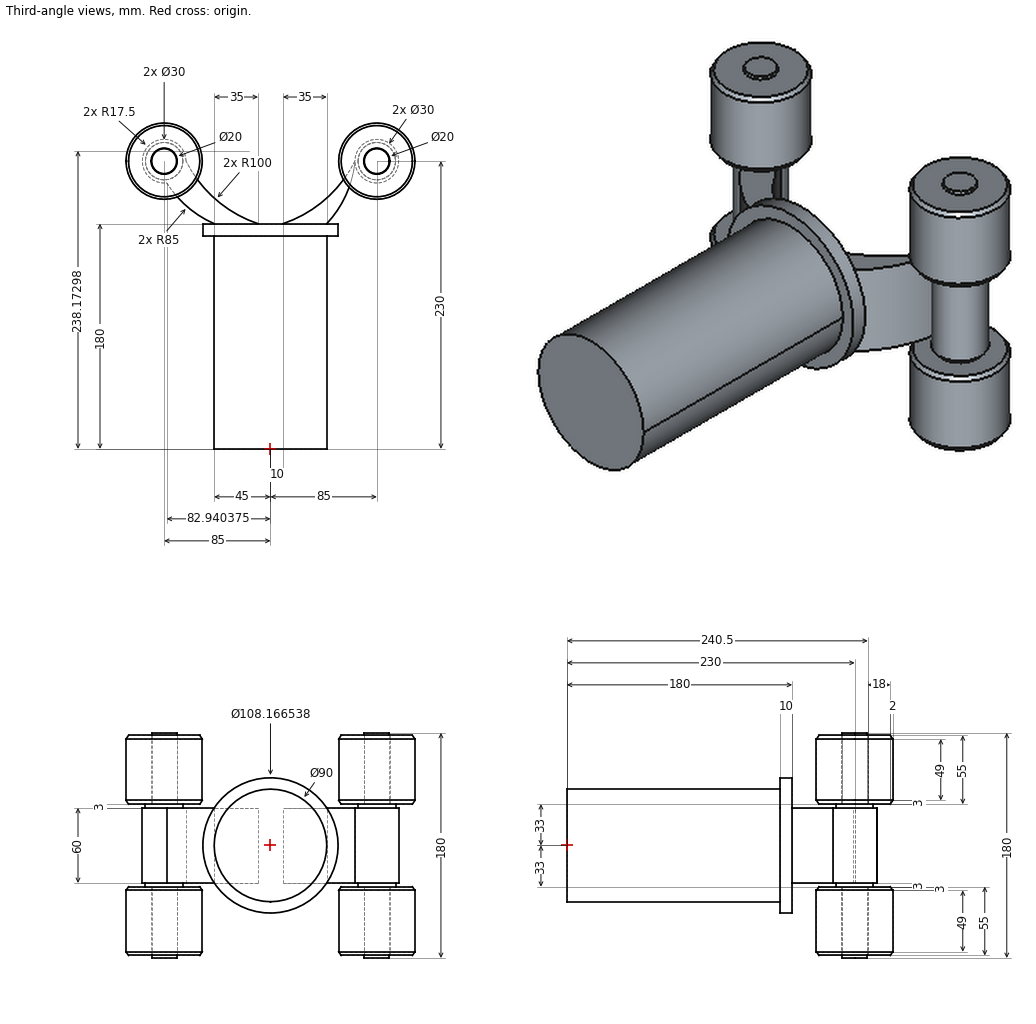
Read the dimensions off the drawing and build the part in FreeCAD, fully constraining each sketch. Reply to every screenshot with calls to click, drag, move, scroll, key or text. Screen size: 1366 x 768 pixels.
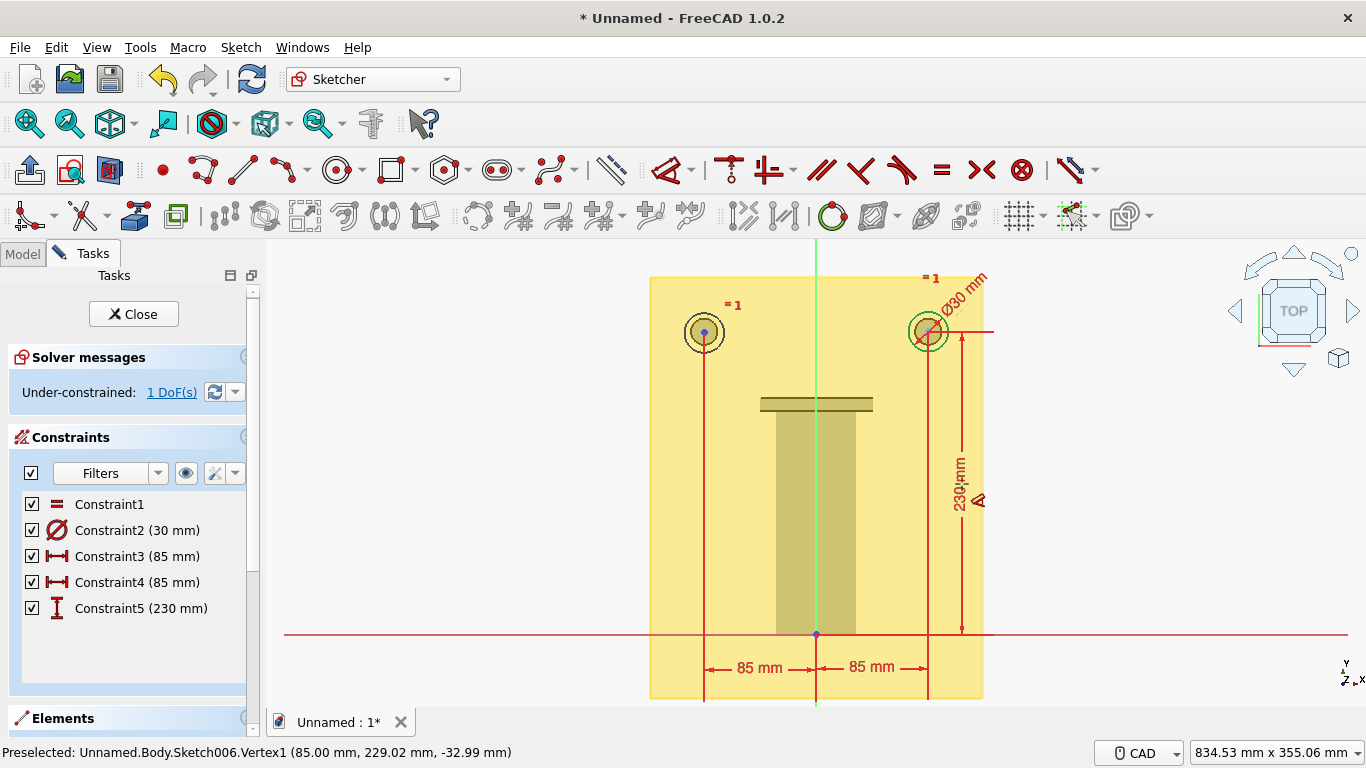
click(704, 333)
click(670, 484)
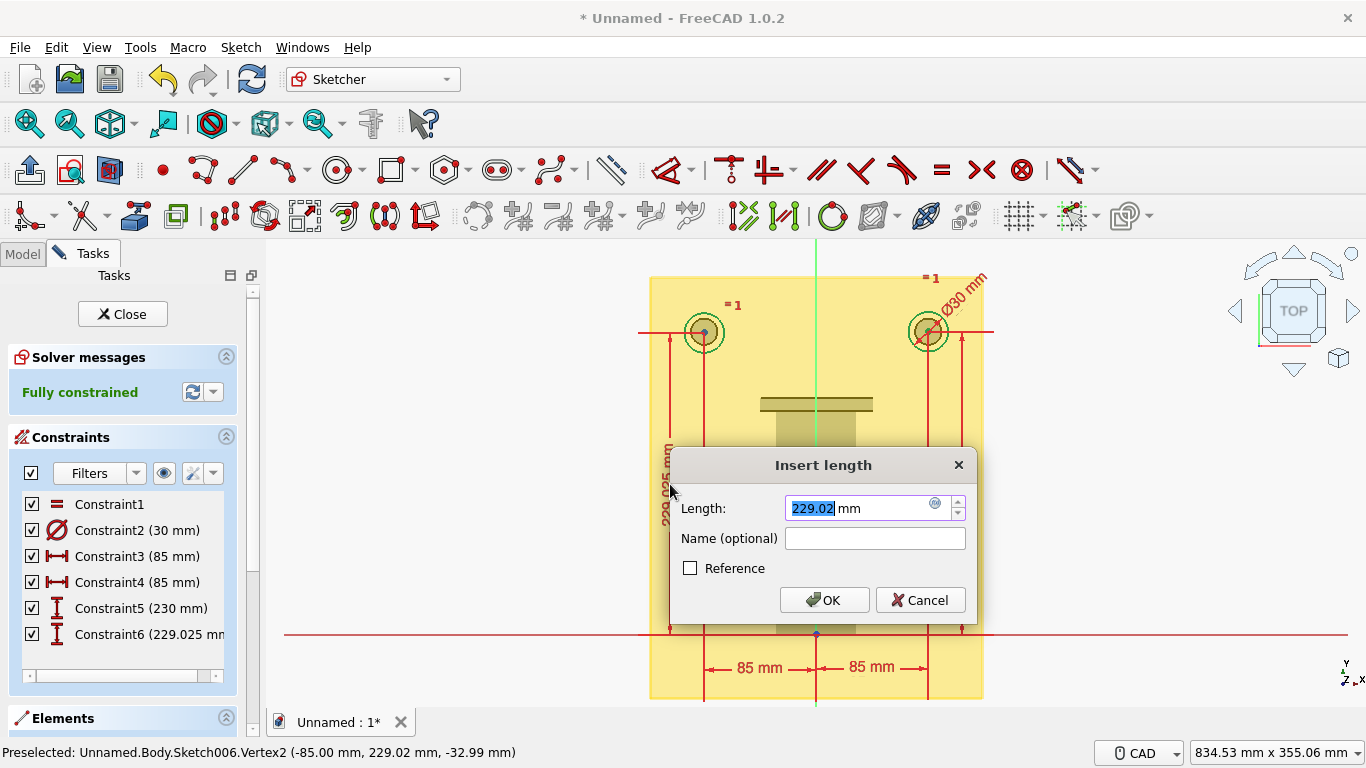
text(230)
key(Return)
key(Escape)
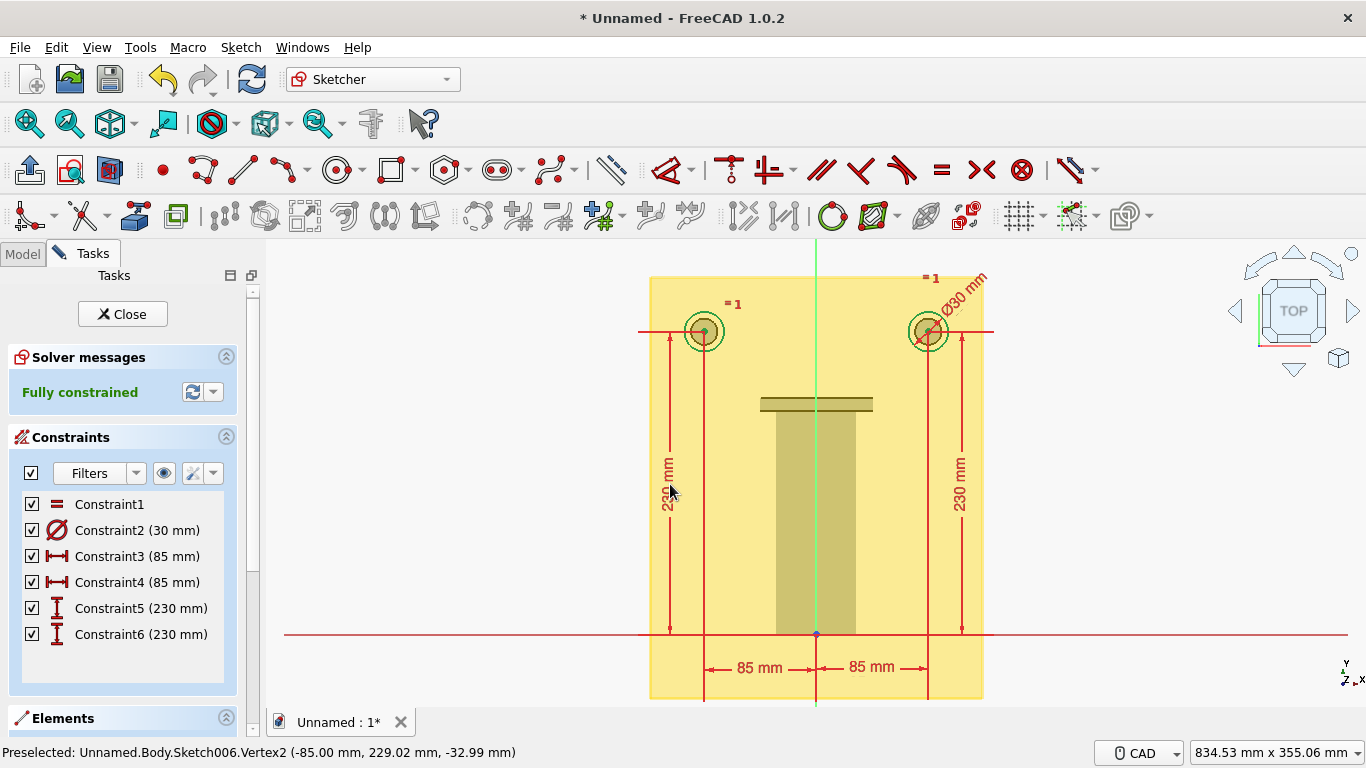
click(123, 314)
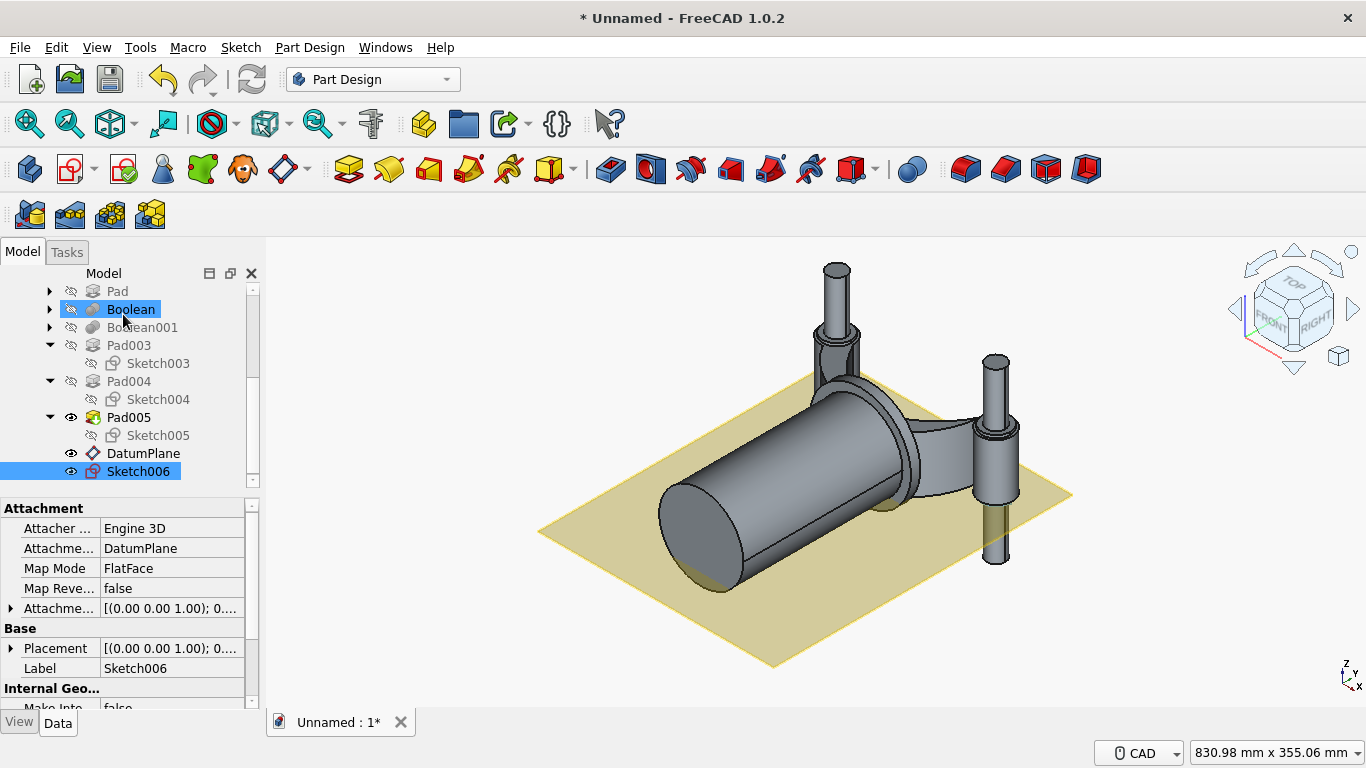
click(350, 170)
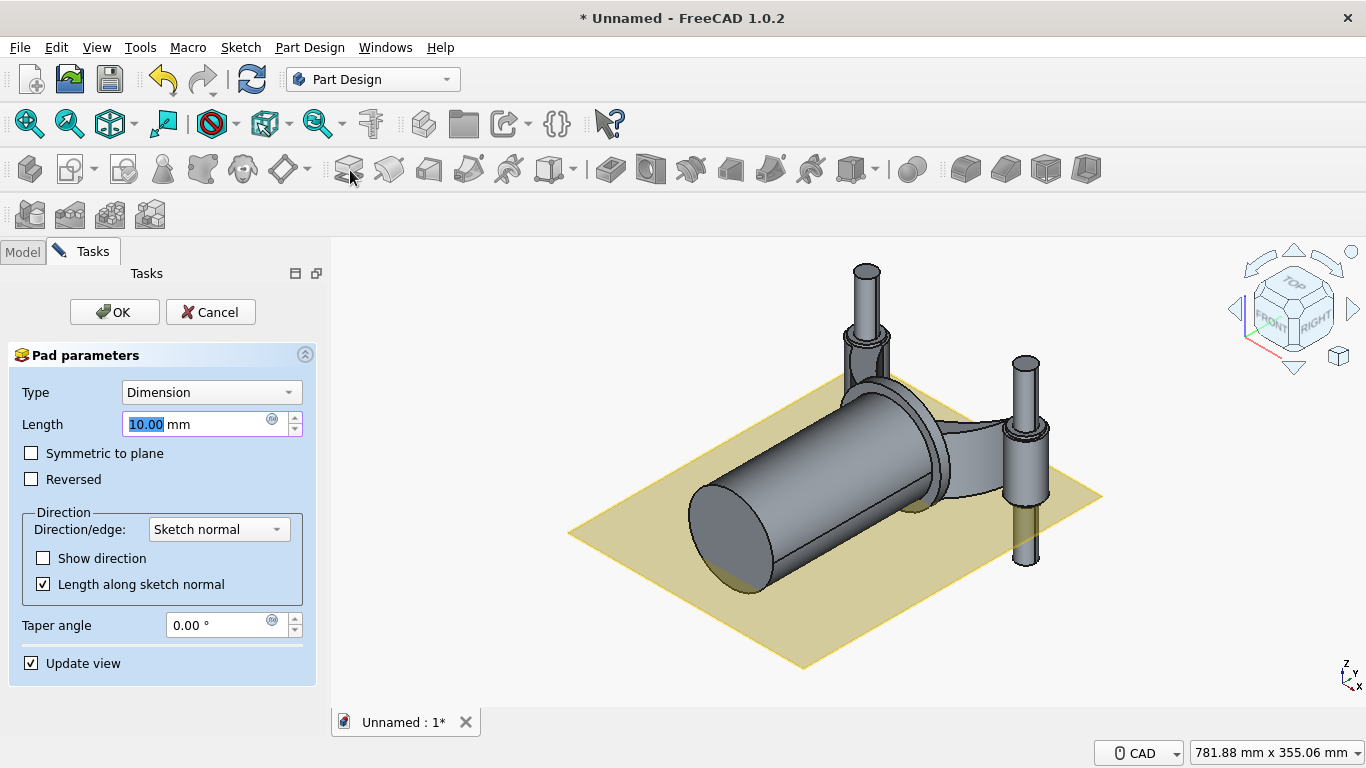
text(3)
key(Tab)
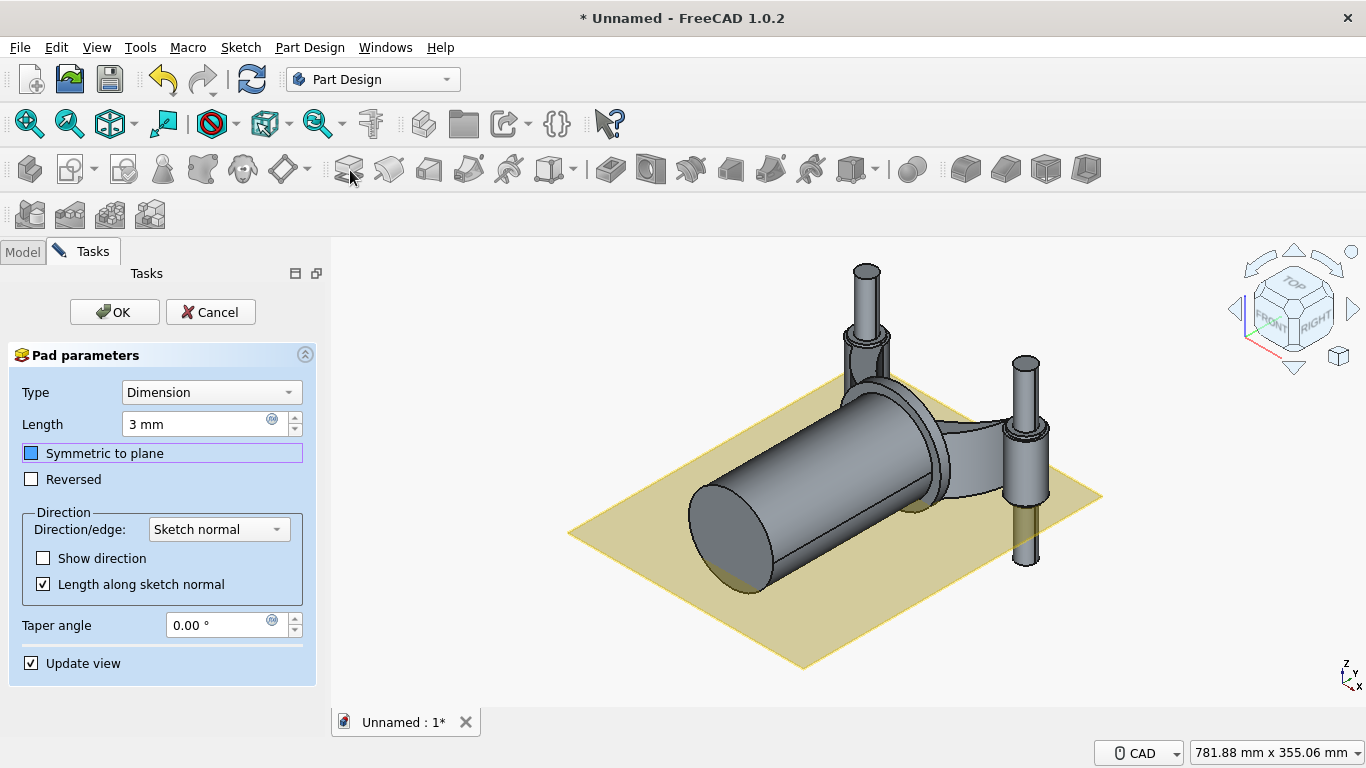
click(115, 312)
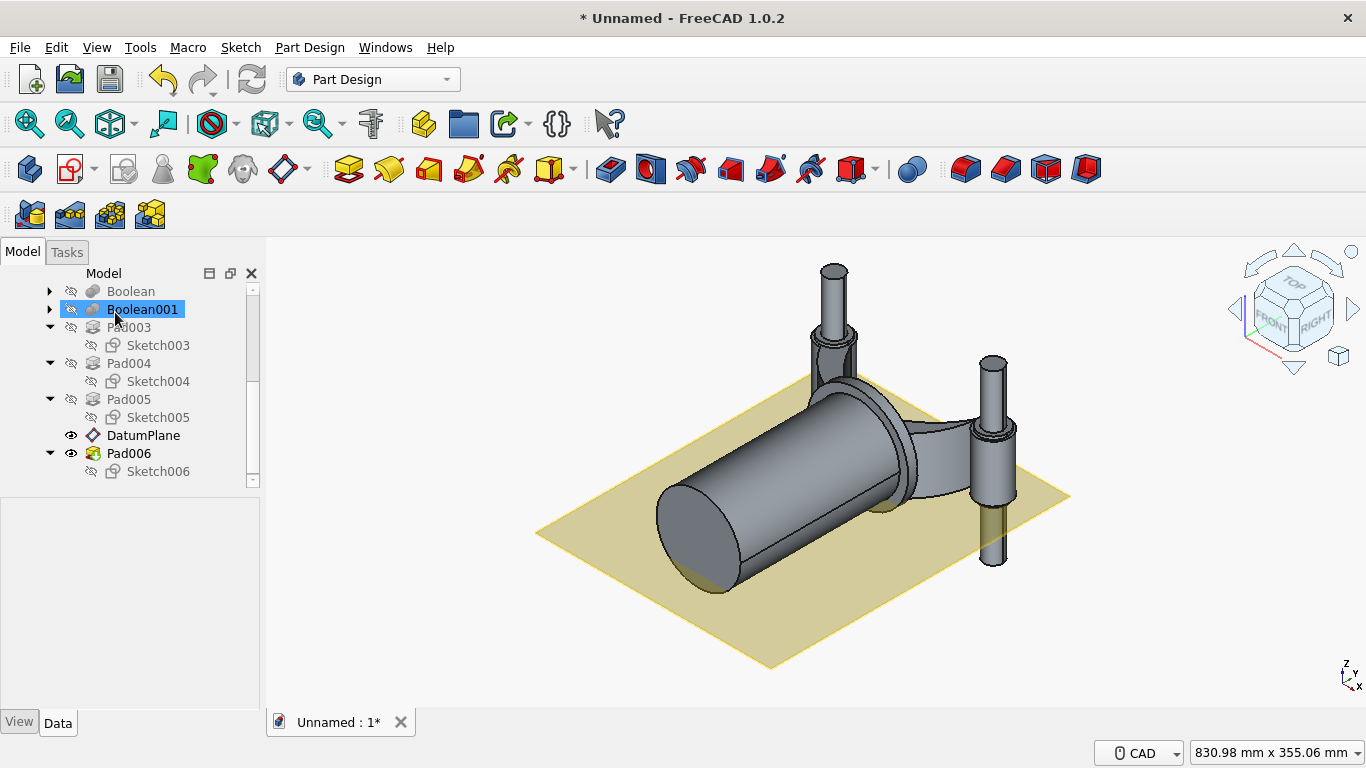
click(116, 435)
key(space)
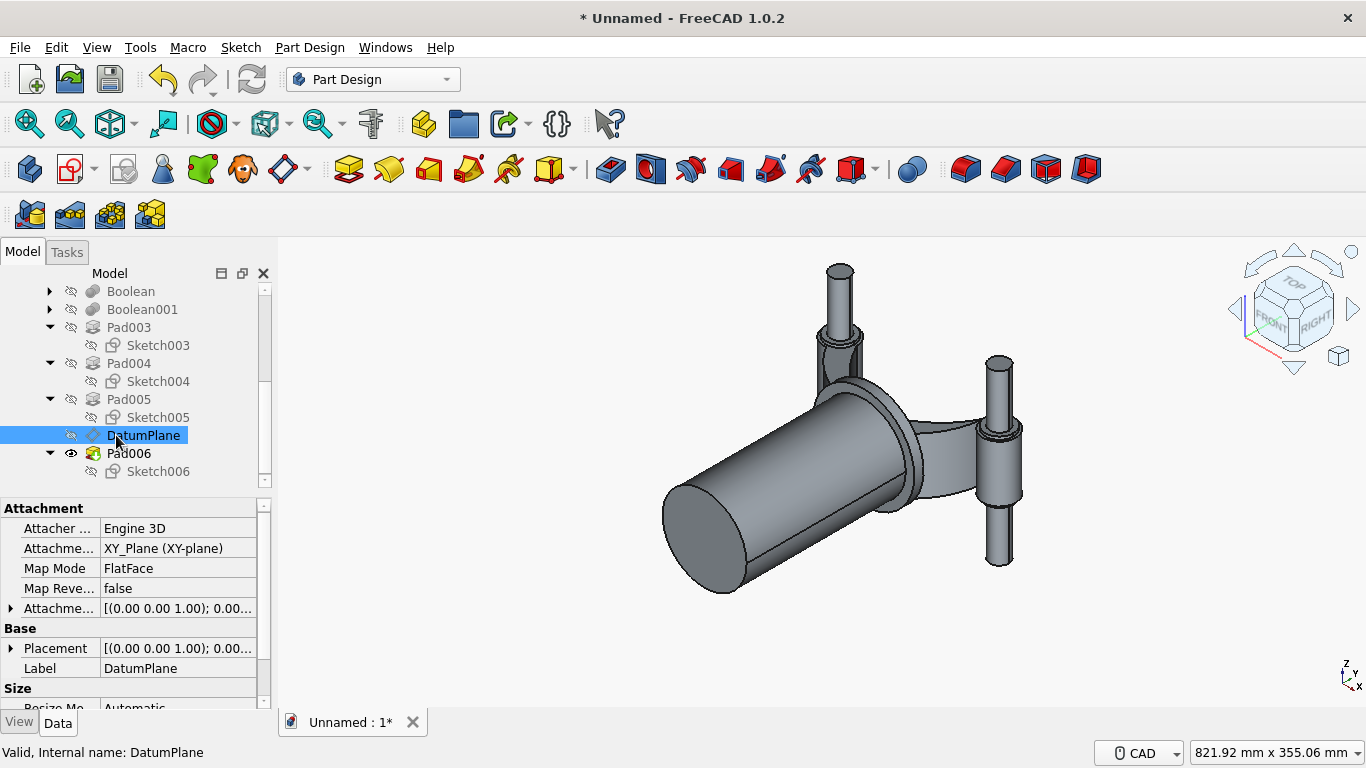
scroll(140, 377, down, 3)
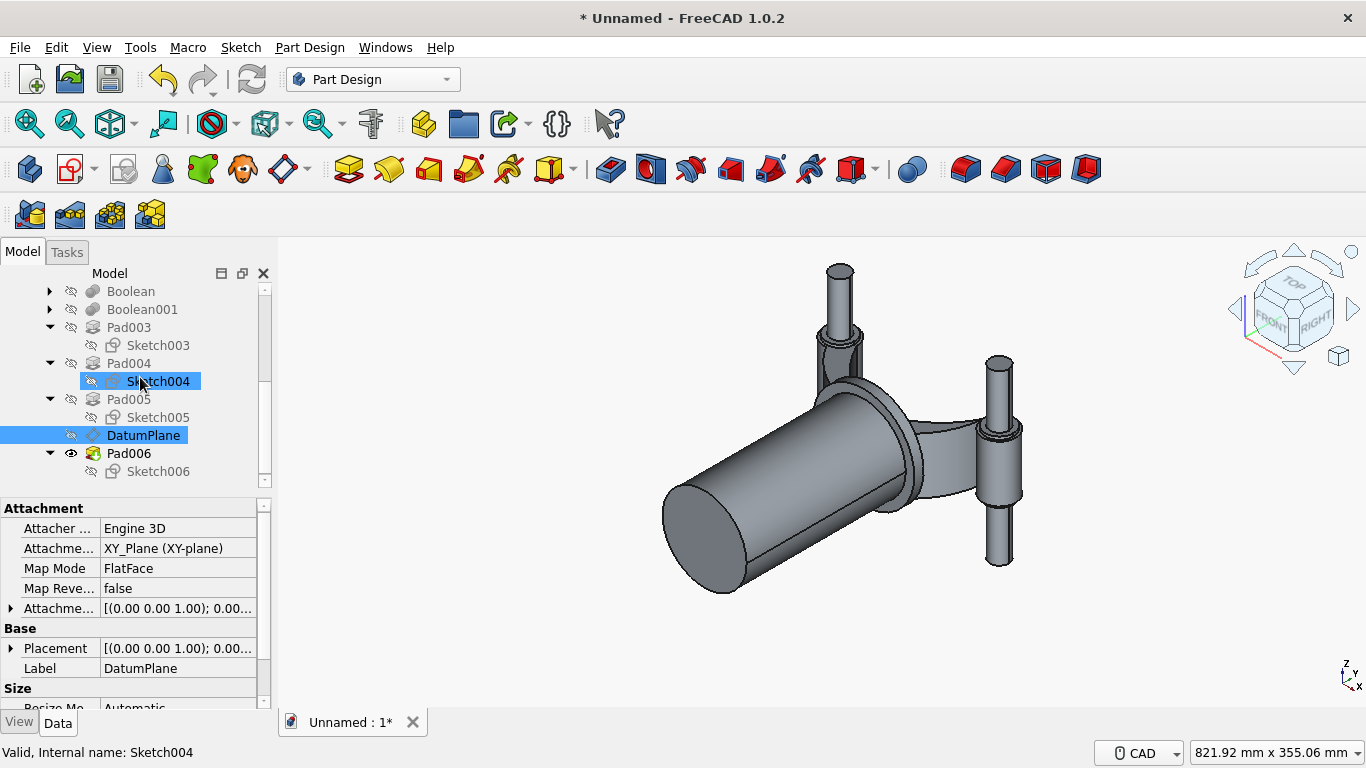
scroll(140, 377, up, 15)